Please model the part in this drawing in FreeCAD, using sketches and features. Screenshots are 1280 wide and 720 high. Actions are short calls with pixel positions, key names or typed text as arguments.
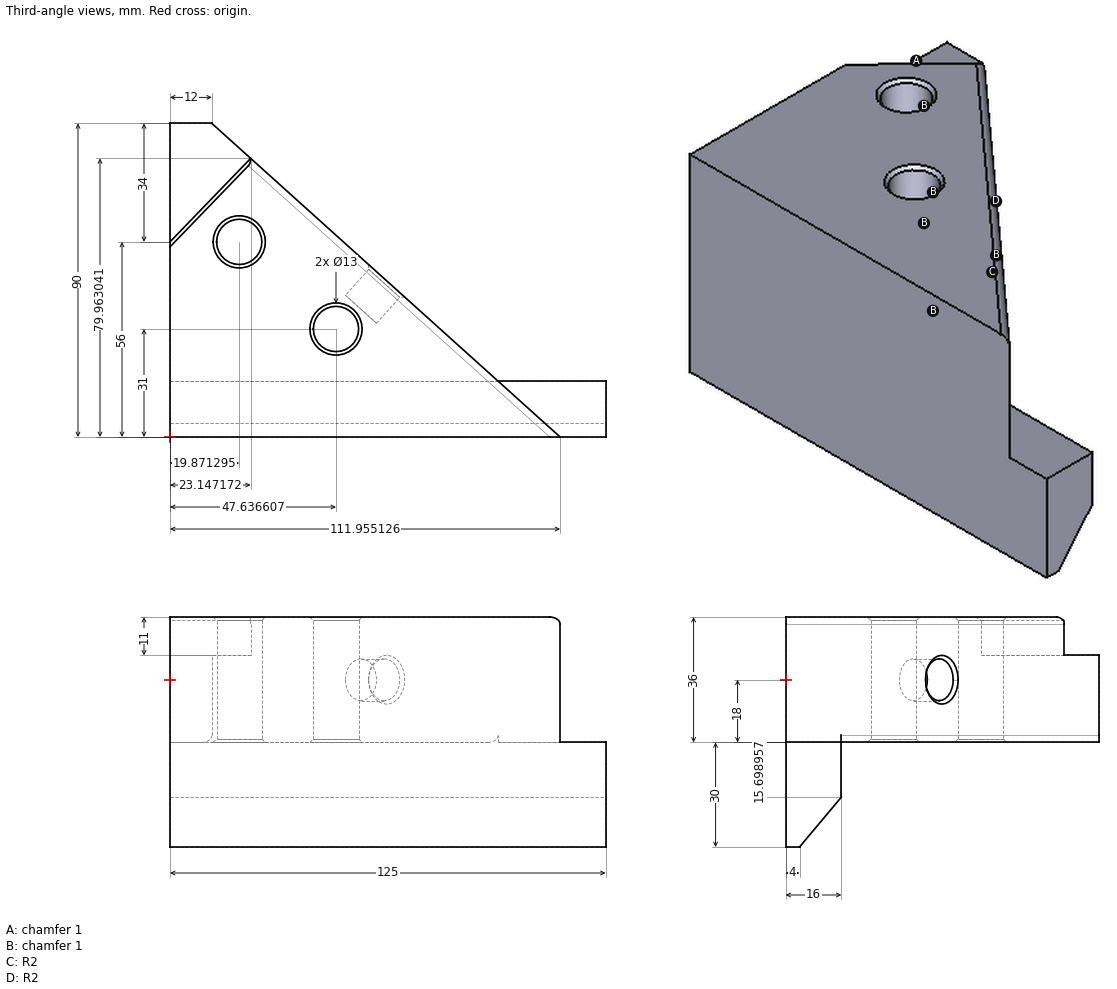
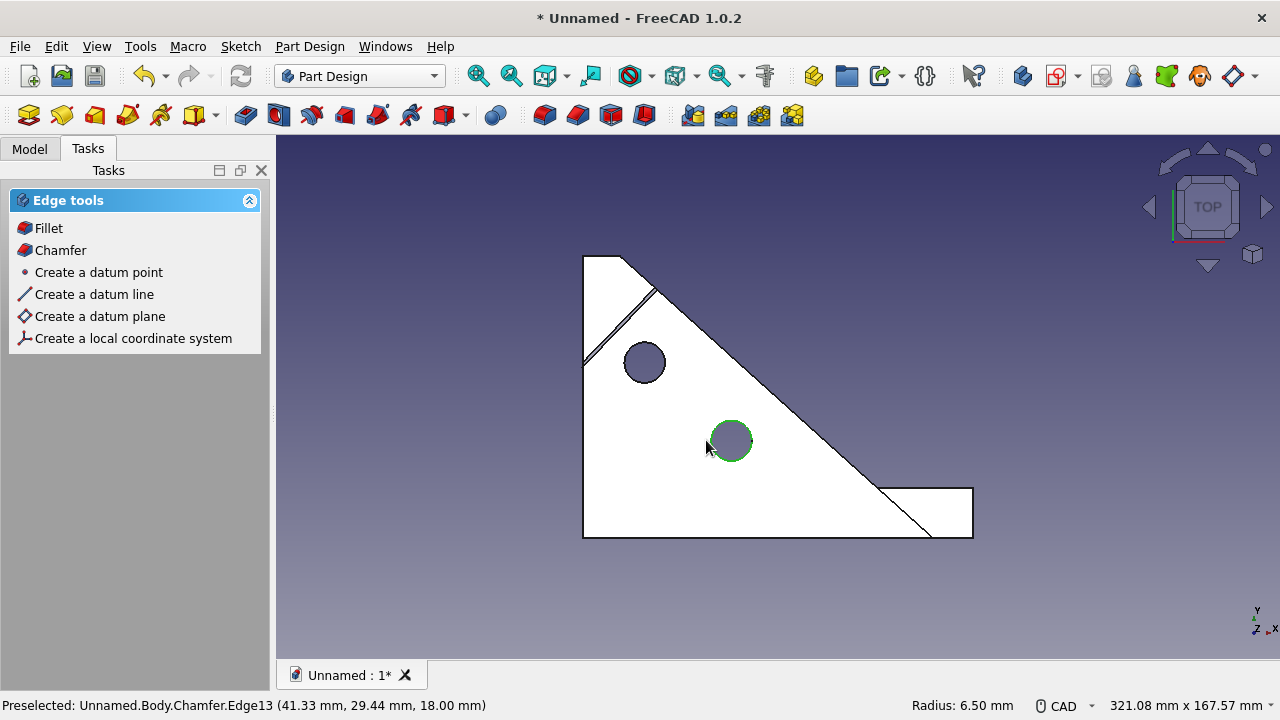
click(624, 362, ctrl)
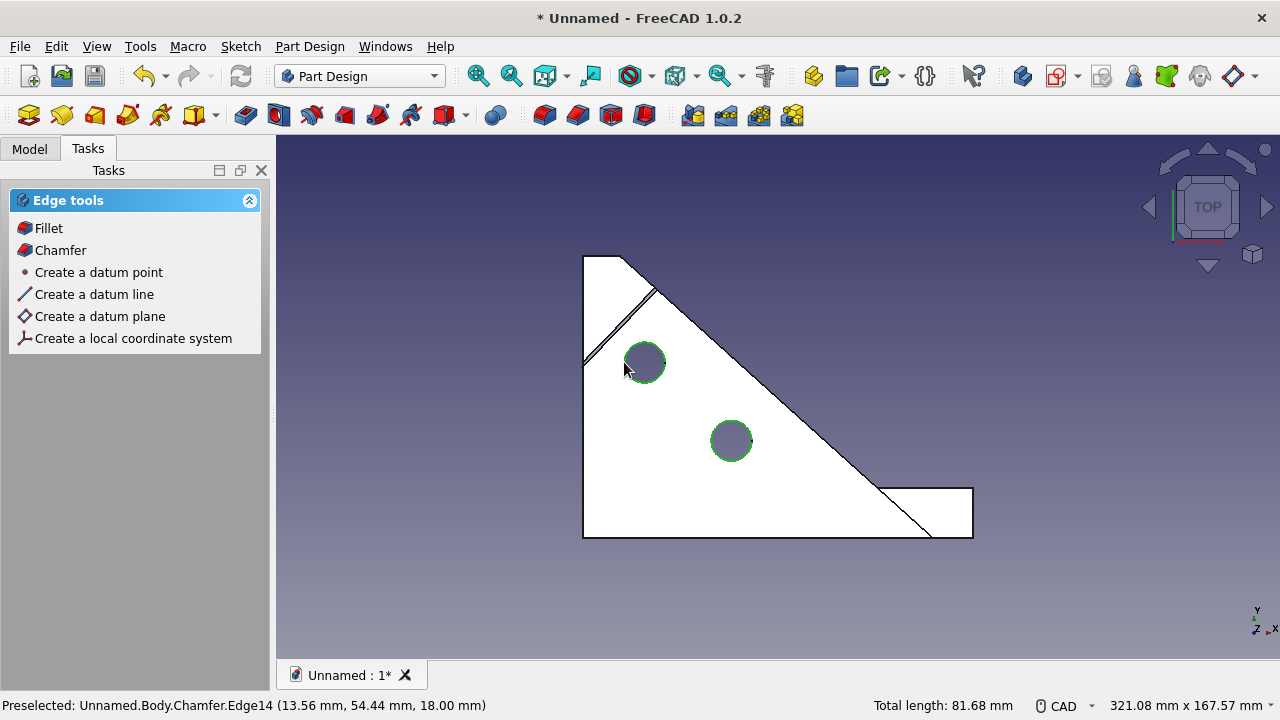
key(0)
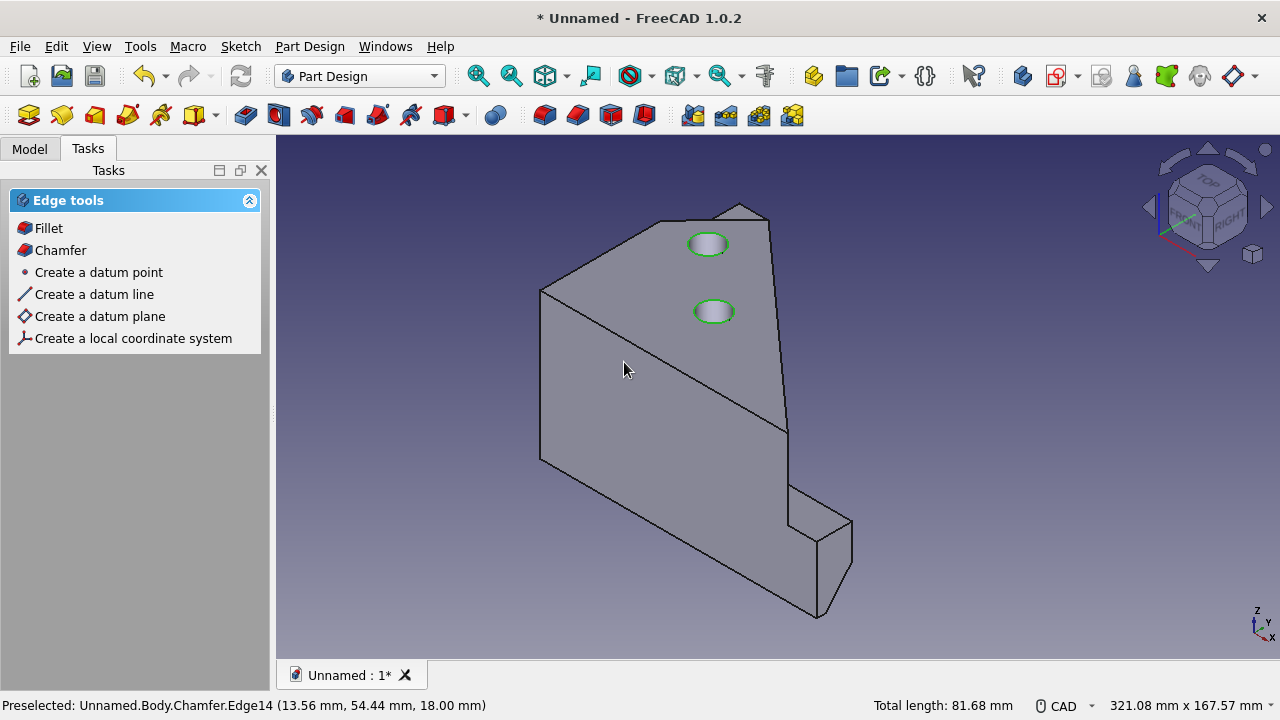
key(2)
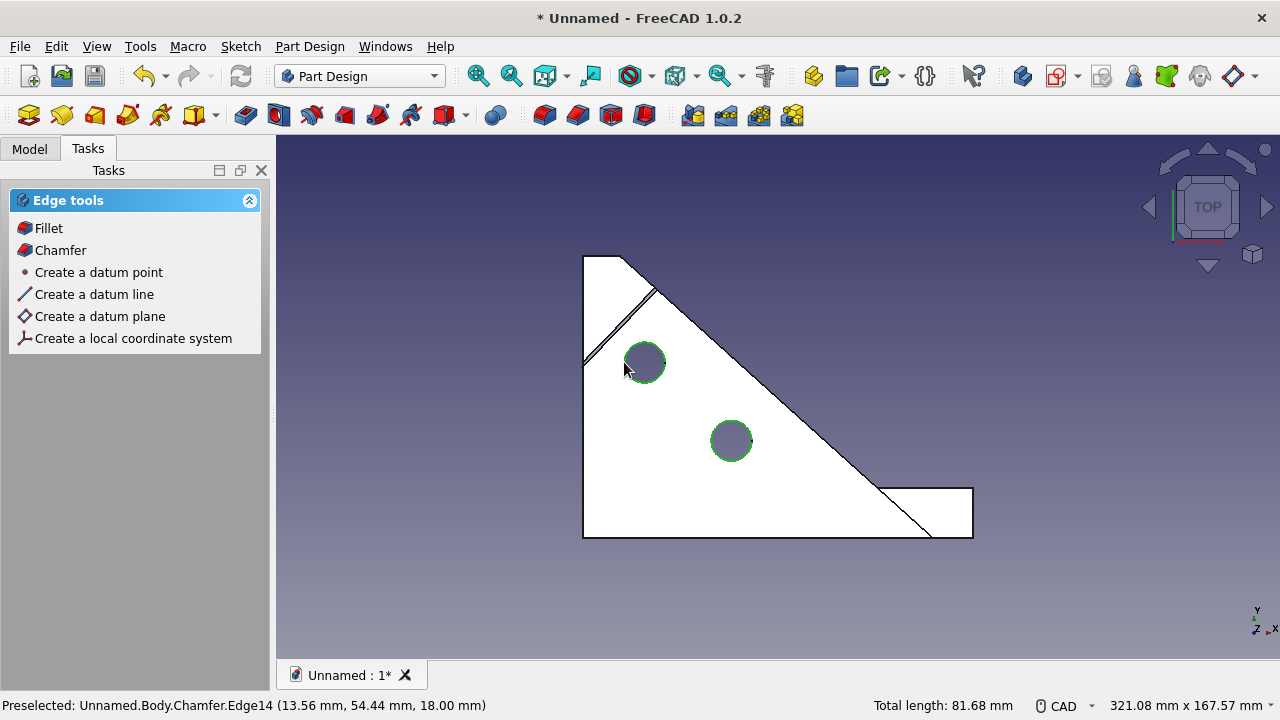
key(1)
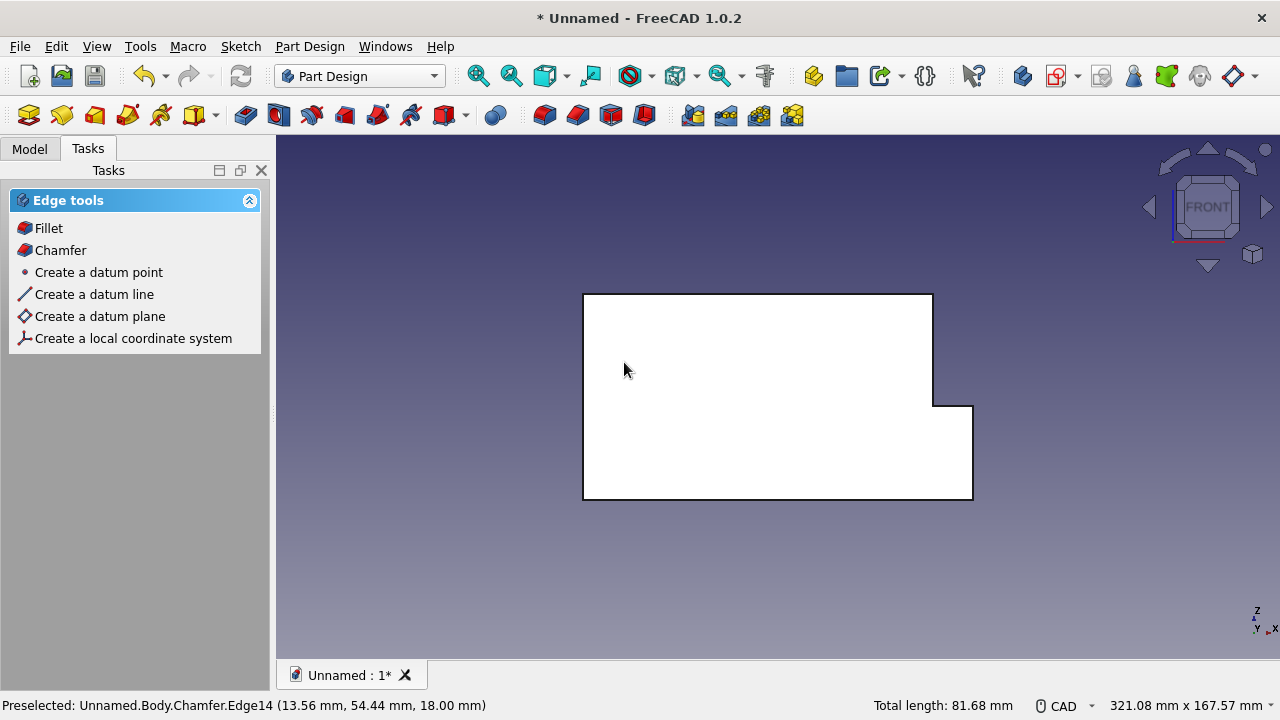
click(479, 76)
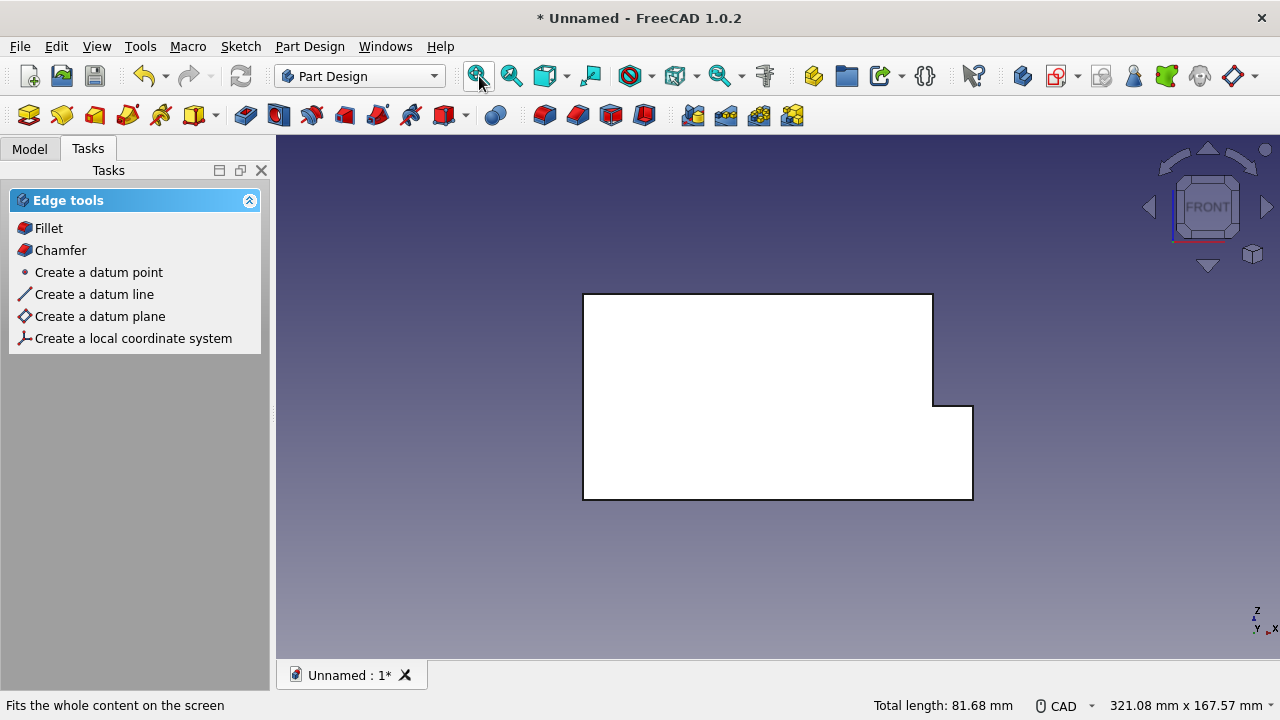
key(3)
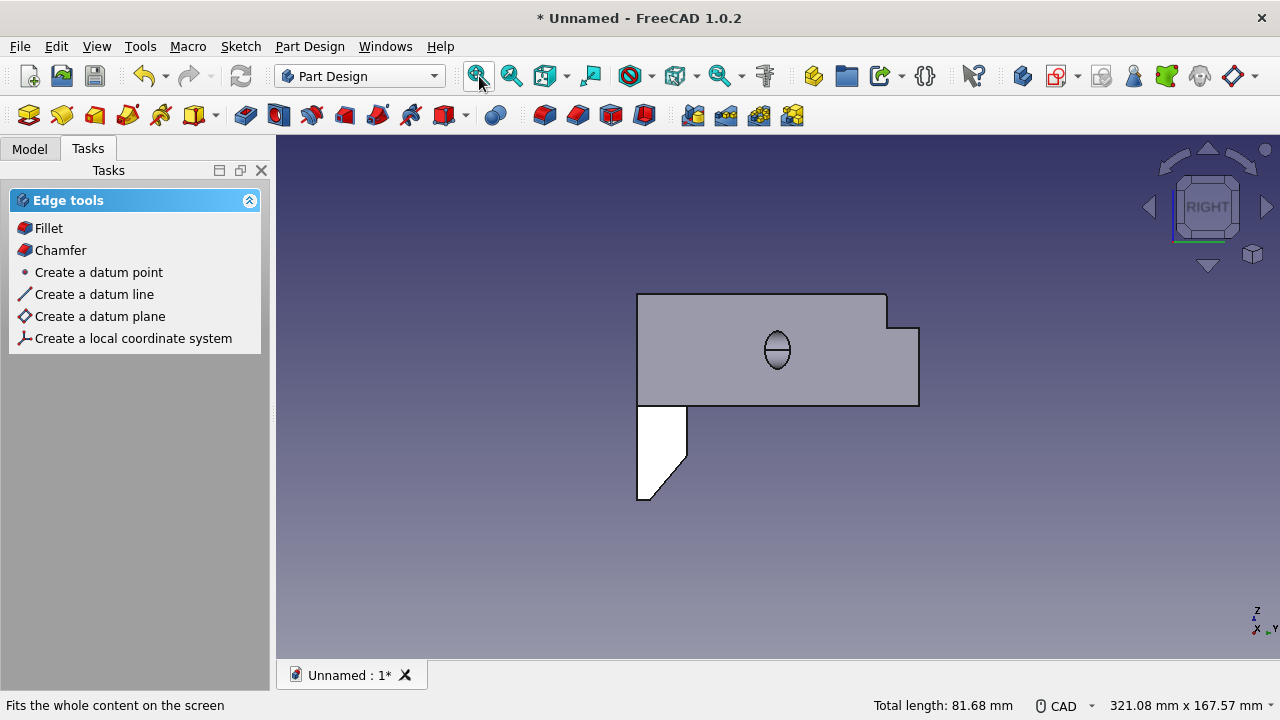
click(479, 76)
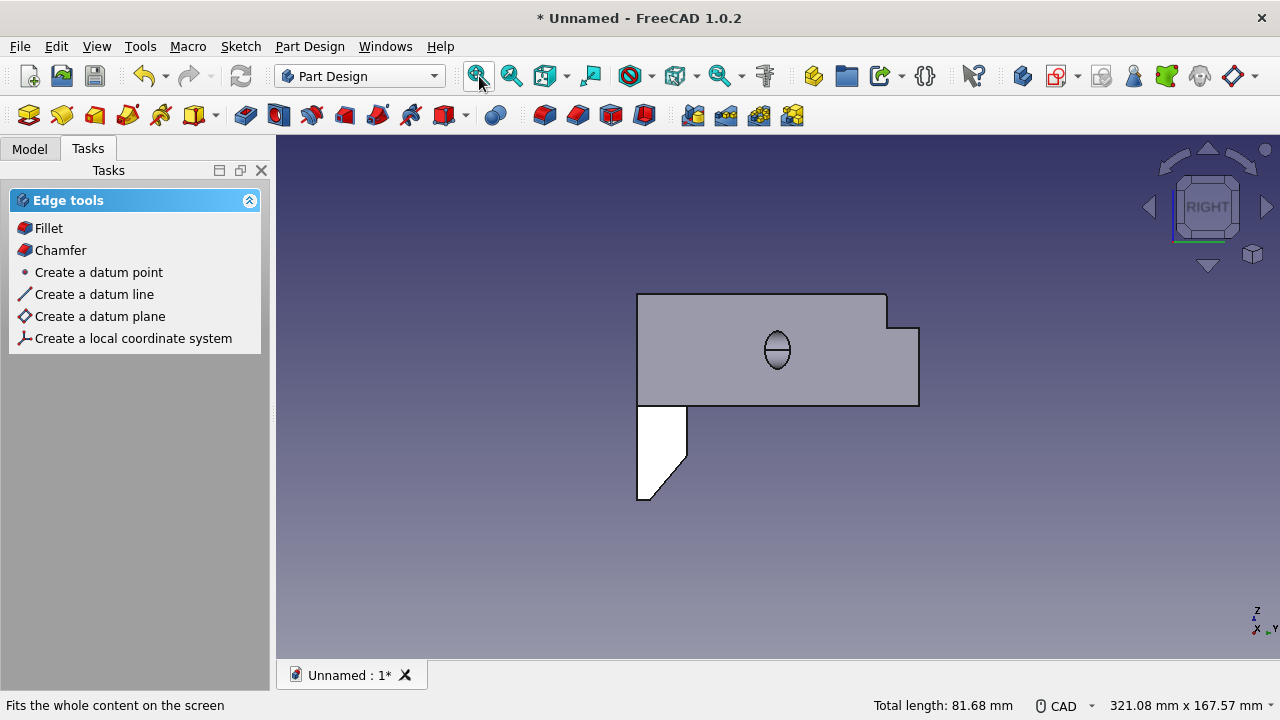
click(781, 331, ctrl)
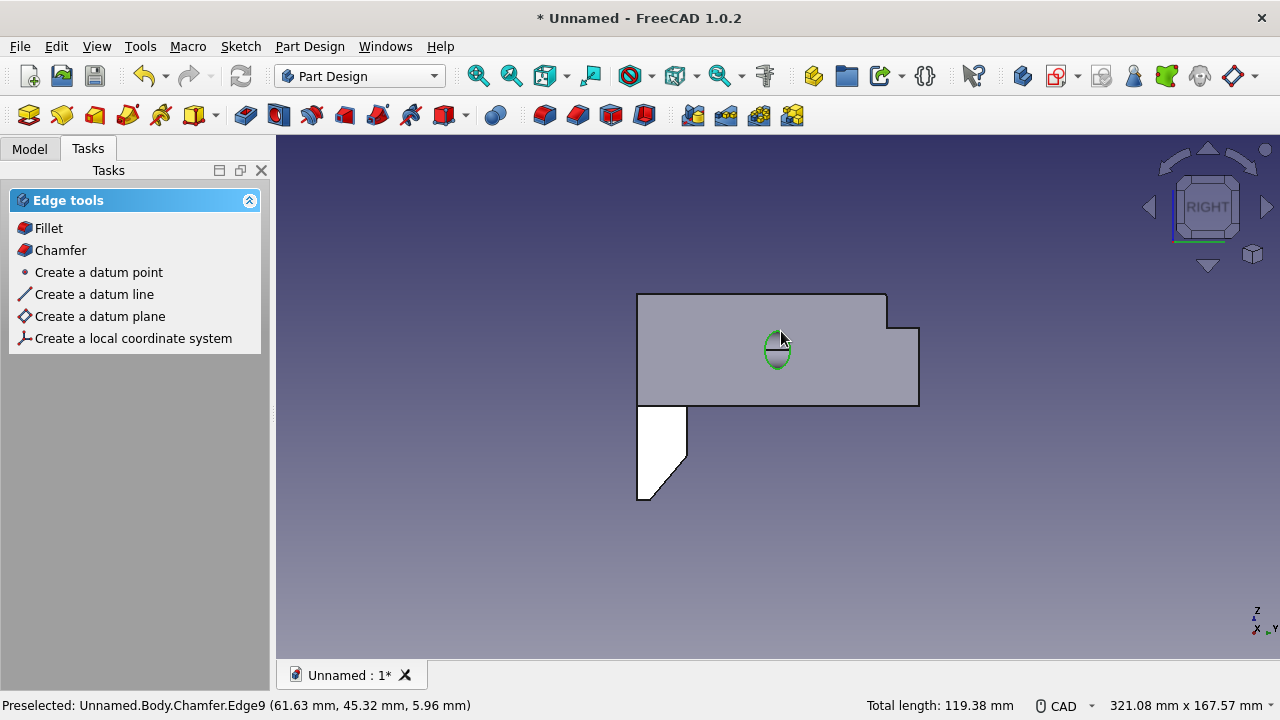
key(5)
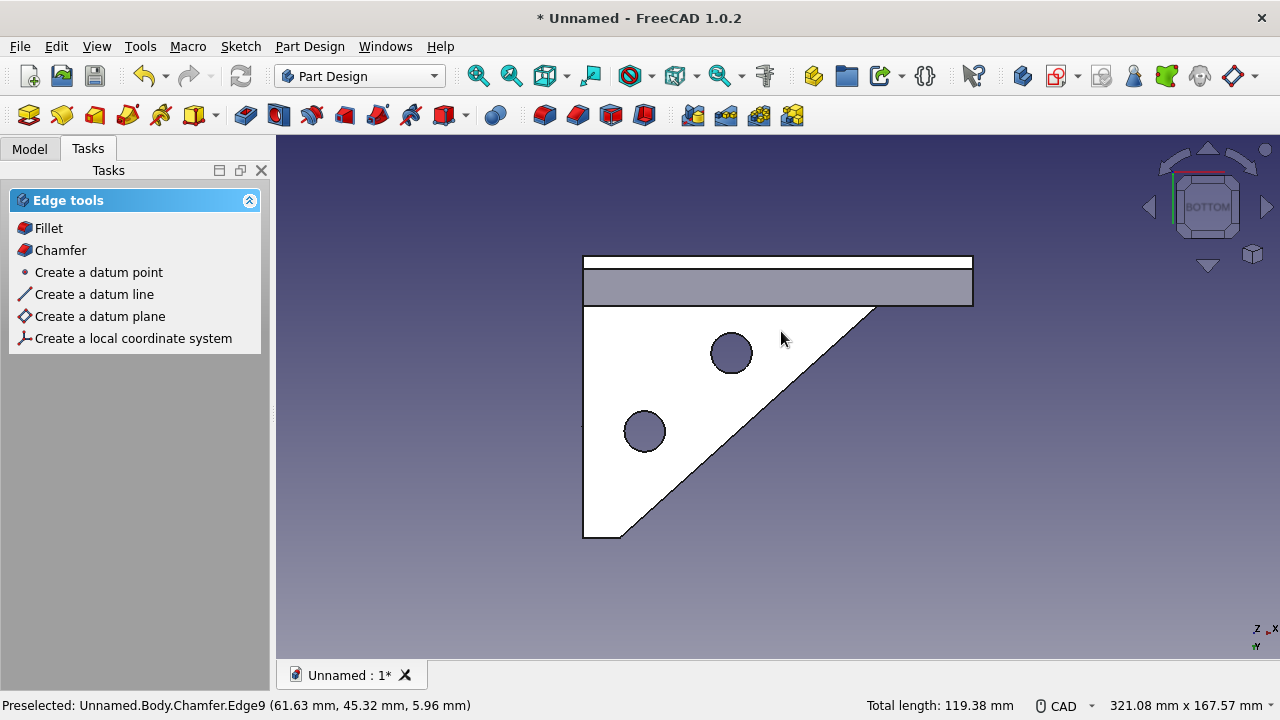
click(711, 352, ctrl)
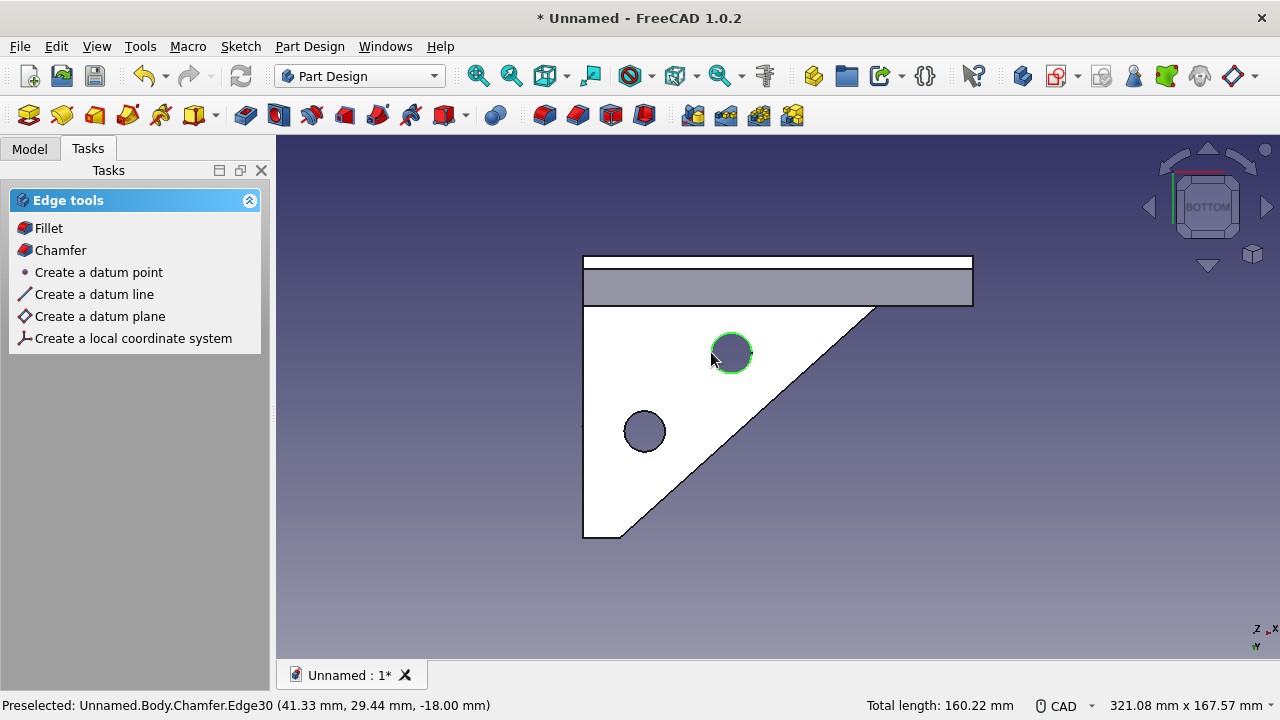
click(624, 430, ctrl)